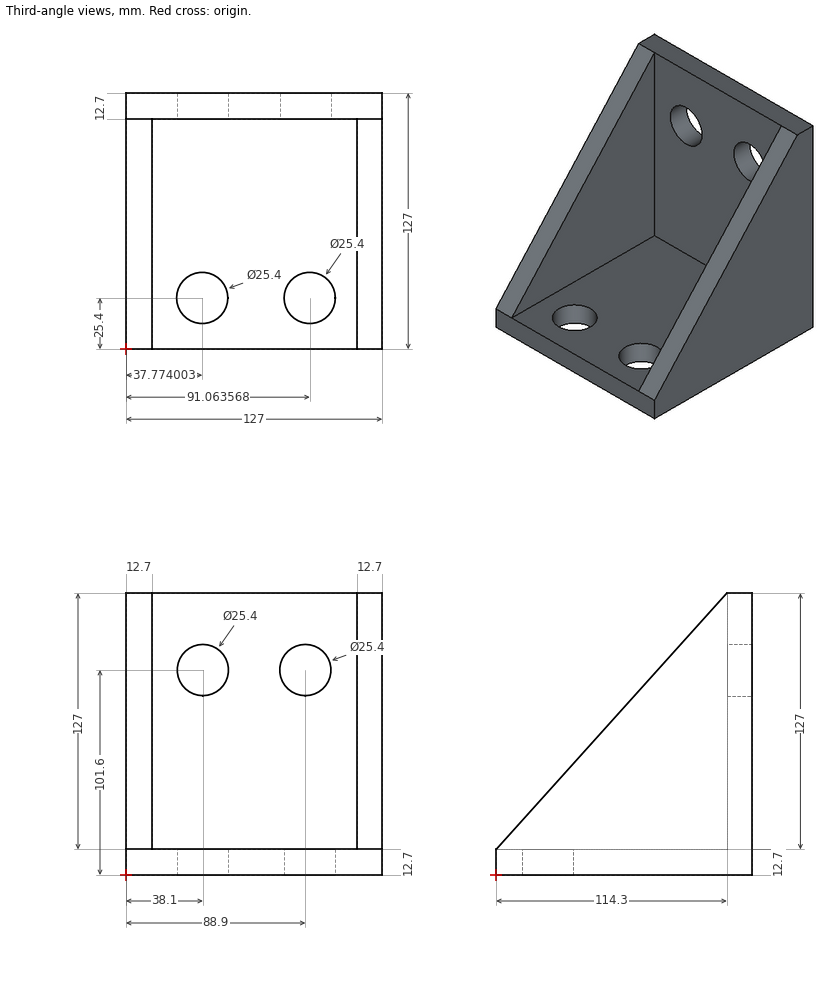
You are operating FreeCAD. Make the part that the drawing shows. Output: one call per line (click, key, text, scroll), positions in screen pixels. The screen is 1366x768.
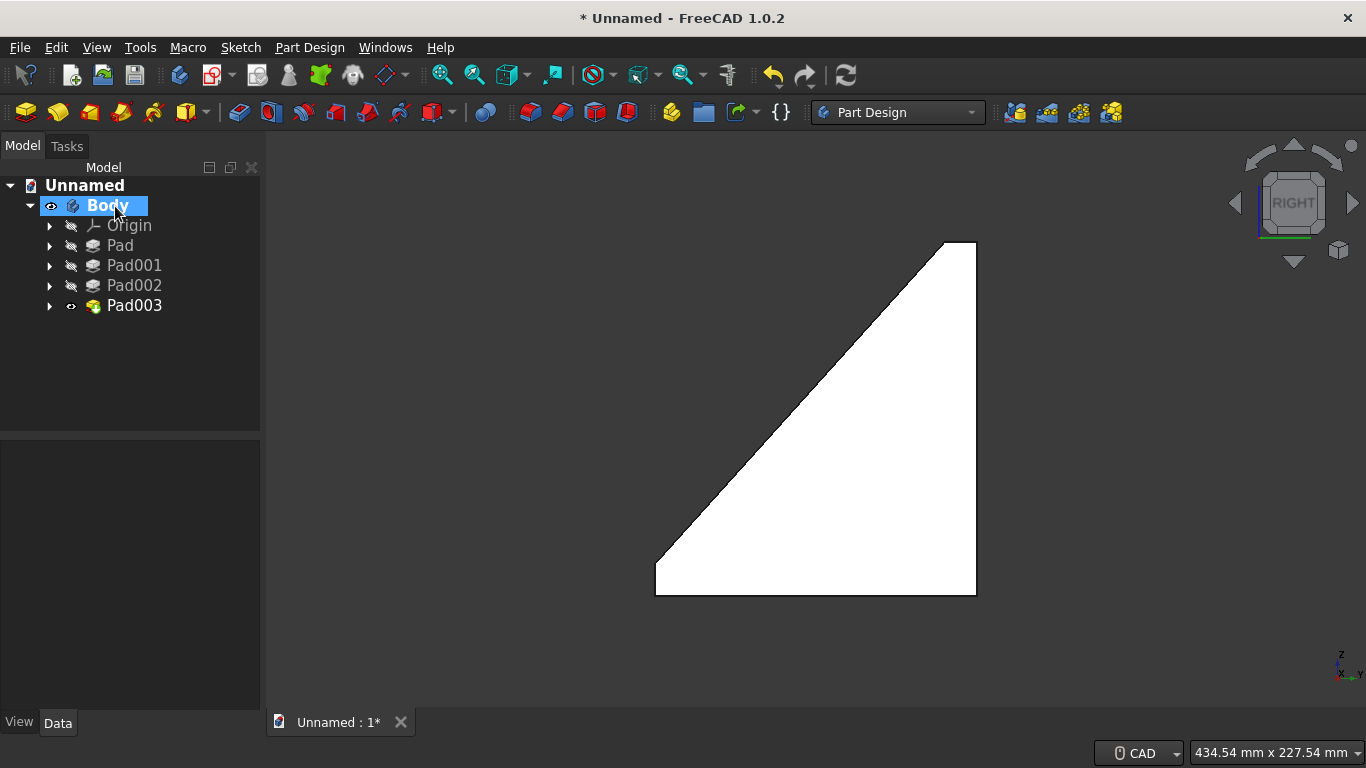
key(0)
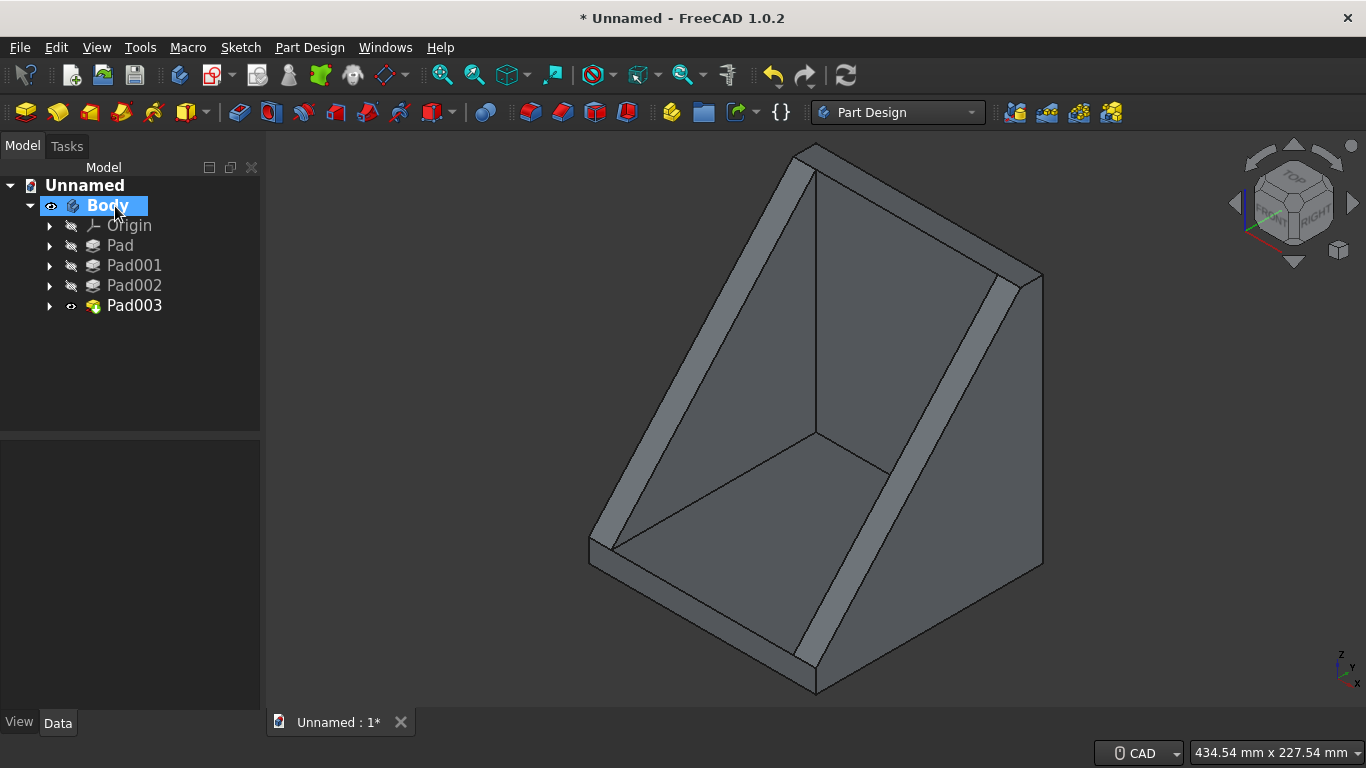
click(907, 352)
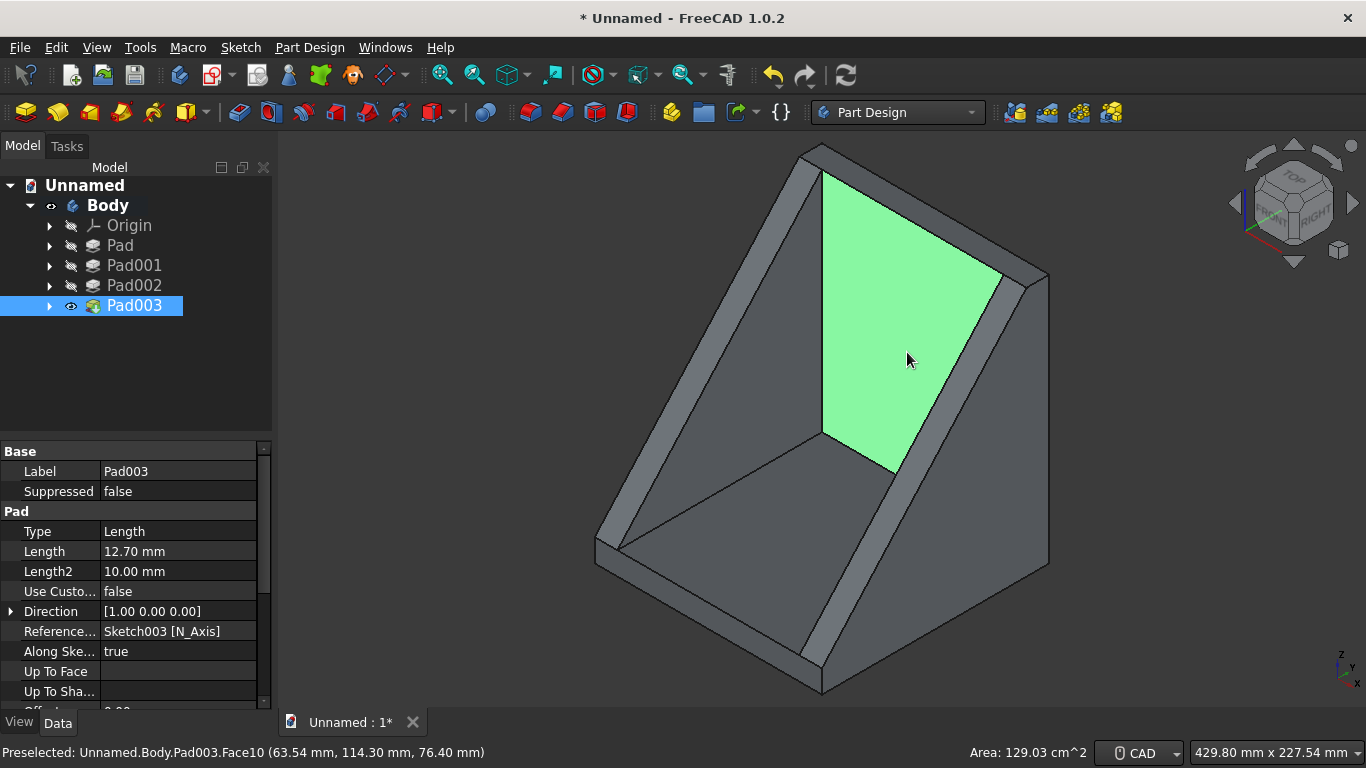
click(212, 76)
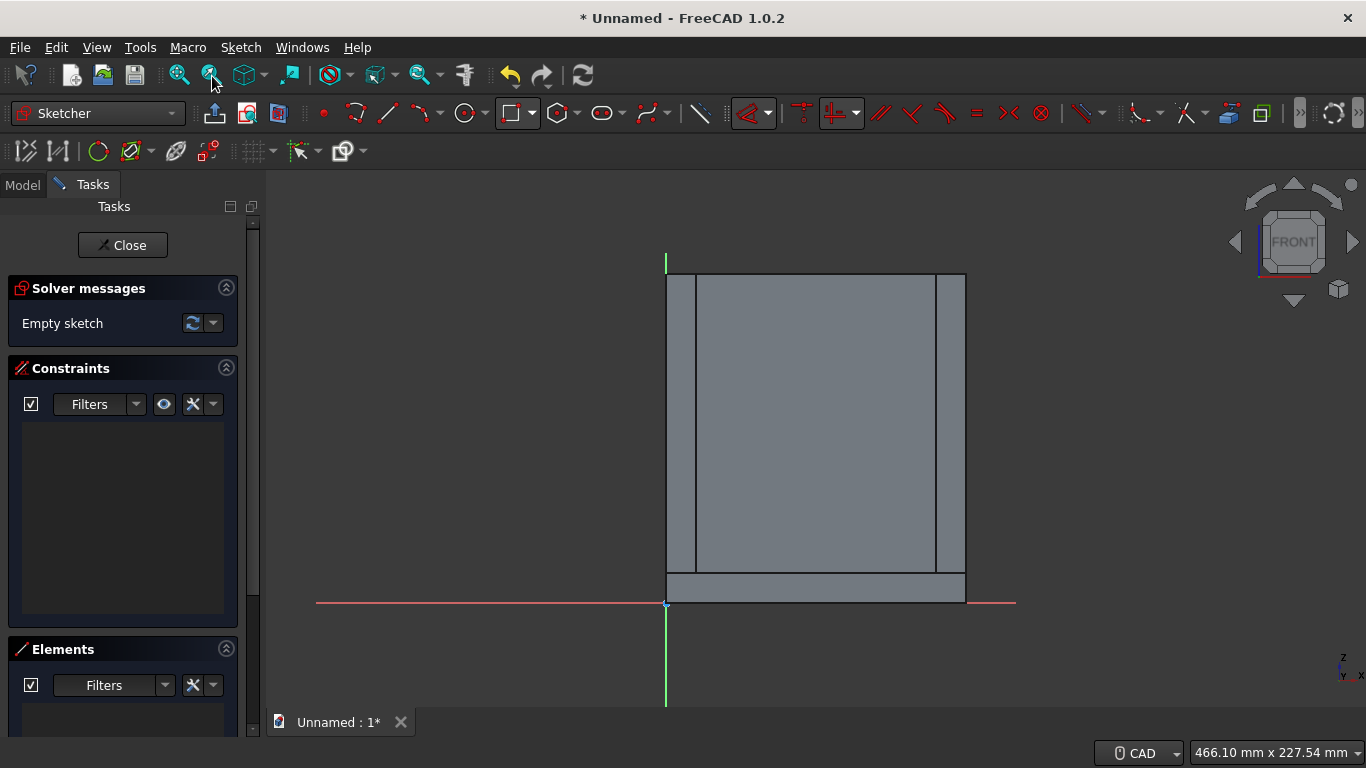
click(280, 114)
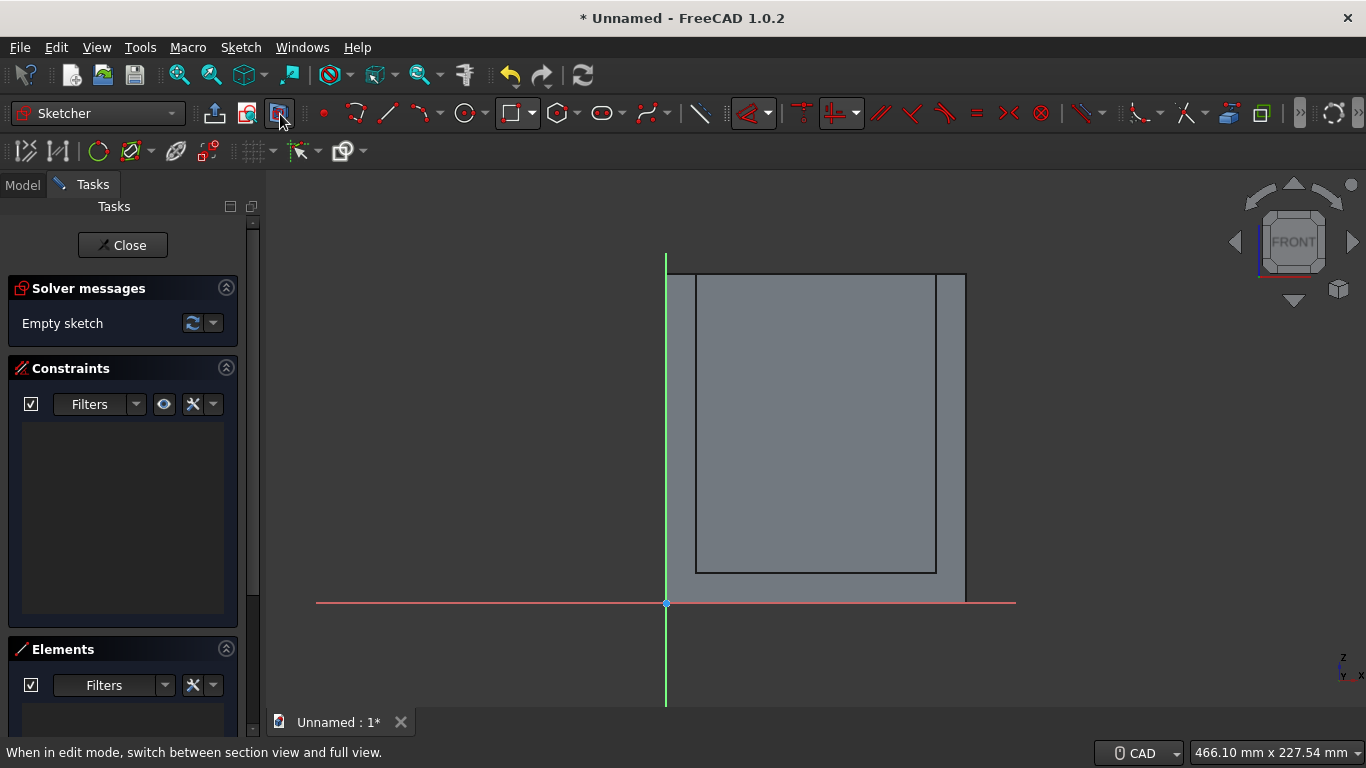
scroll(758, 349, up, 9)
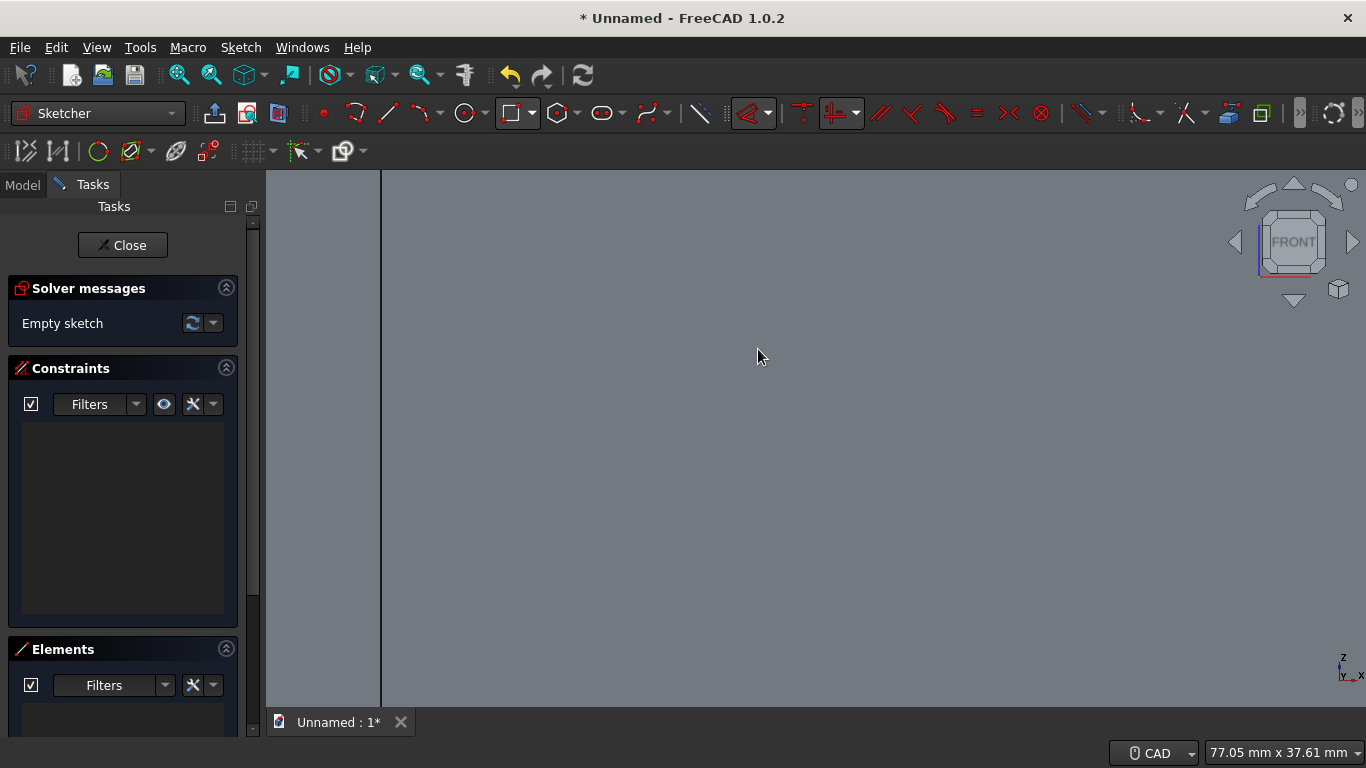
key(g)
key(c)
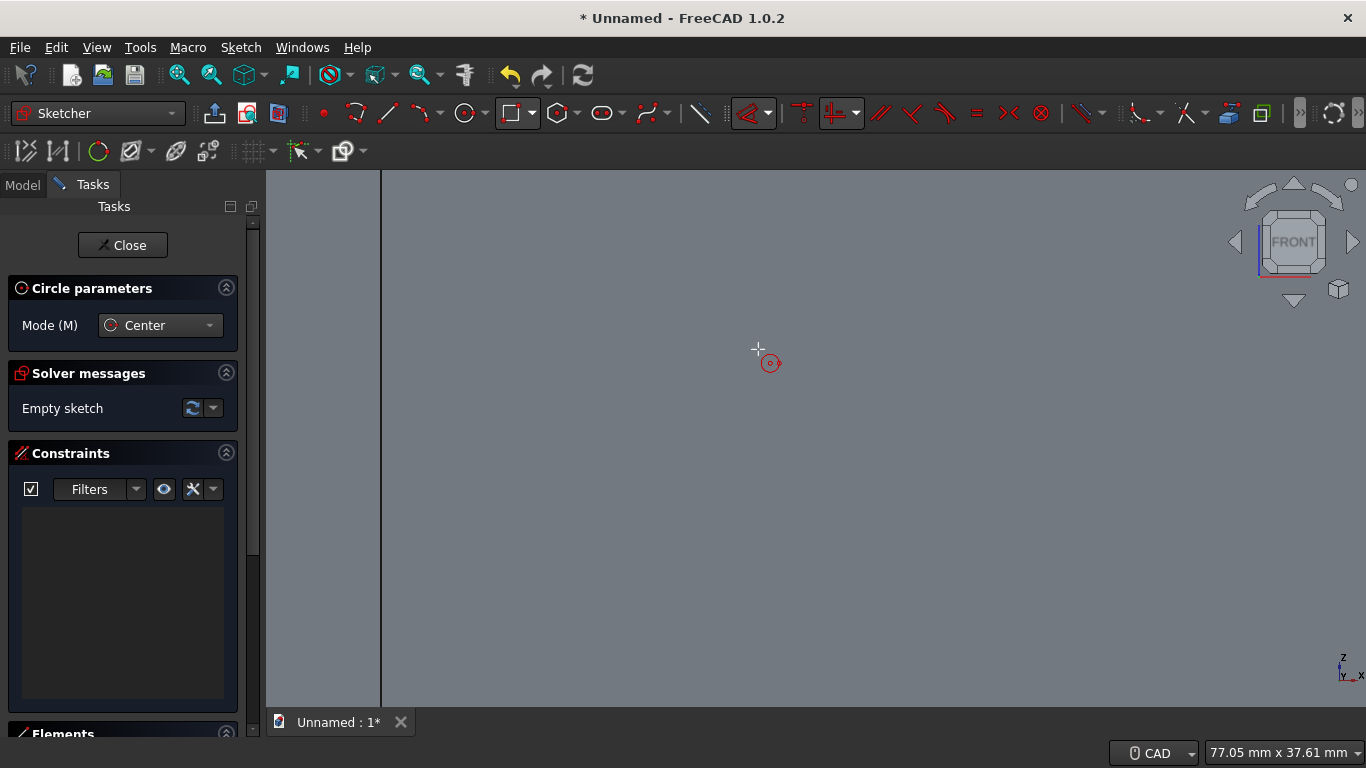
click(744, 435)
click(872, 307)
key(Escape)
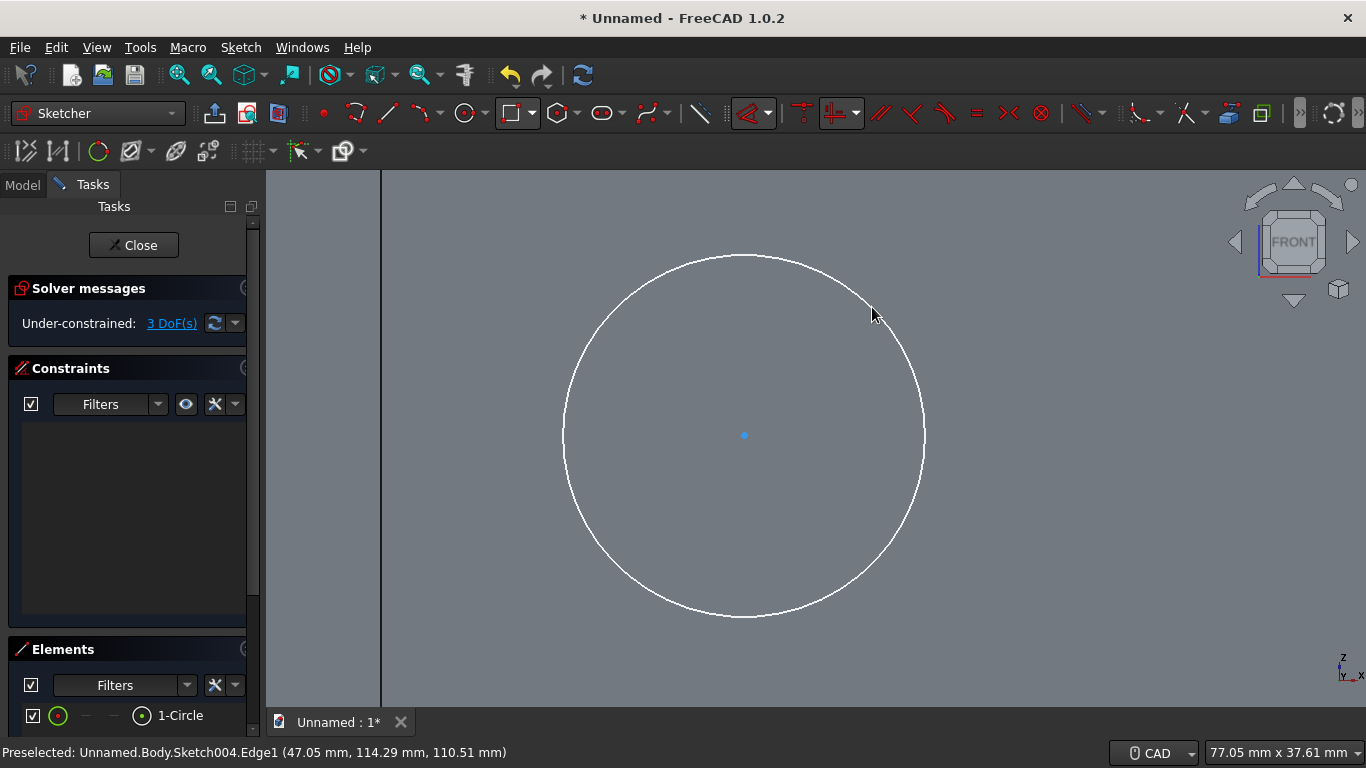
click(872, 308)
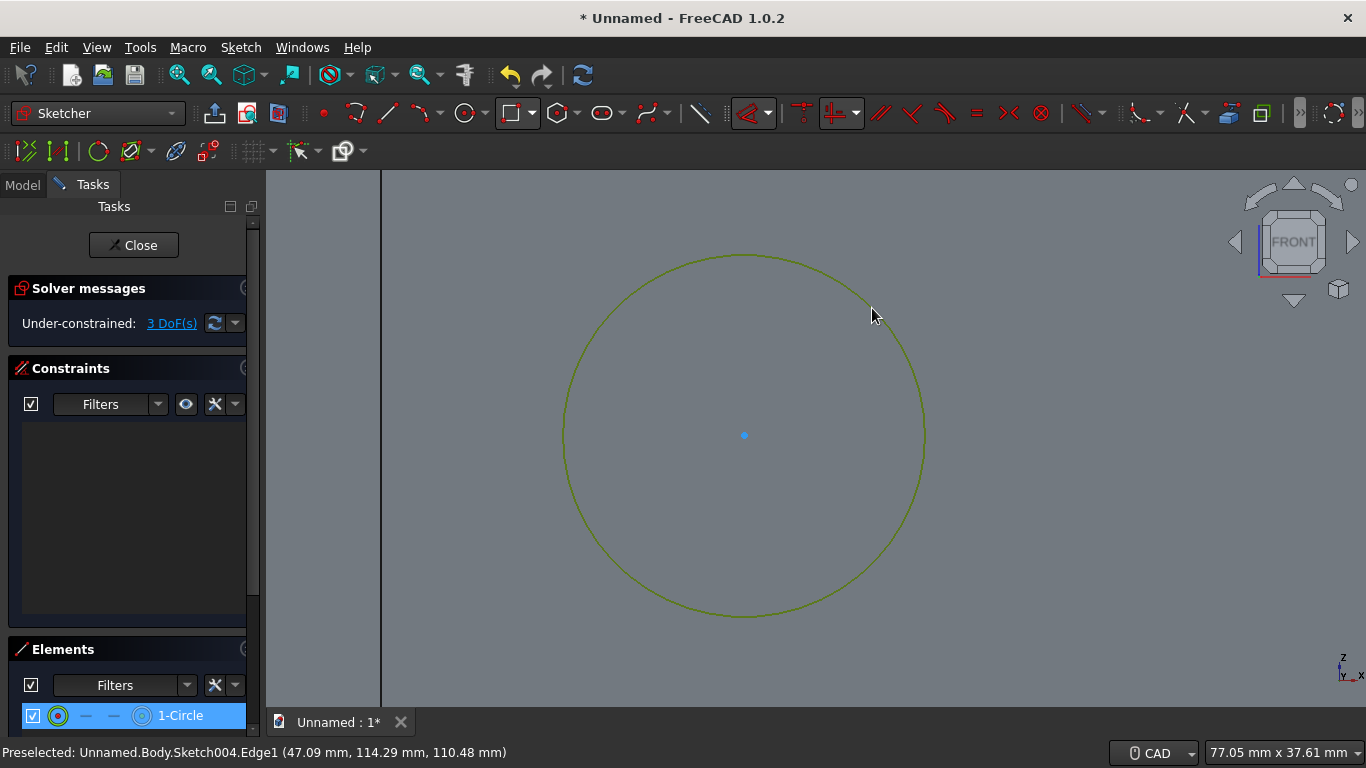
key(k)
key(o)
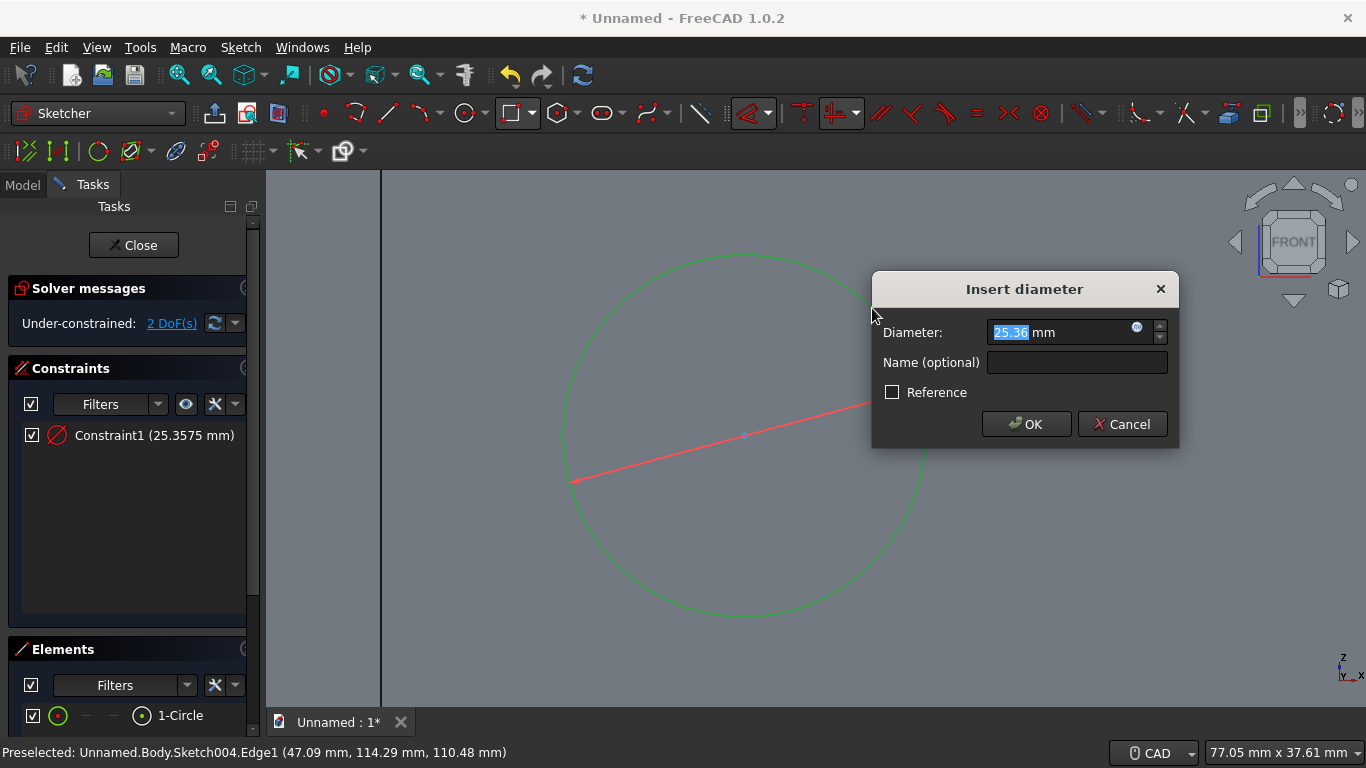
text(25.4)
key(Return)